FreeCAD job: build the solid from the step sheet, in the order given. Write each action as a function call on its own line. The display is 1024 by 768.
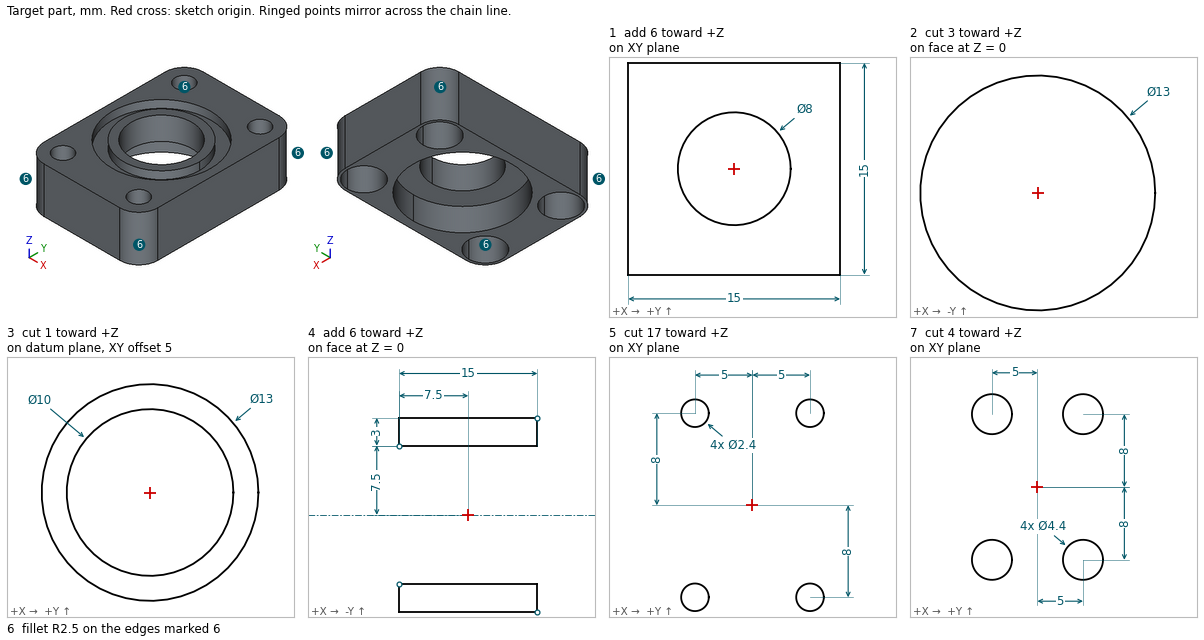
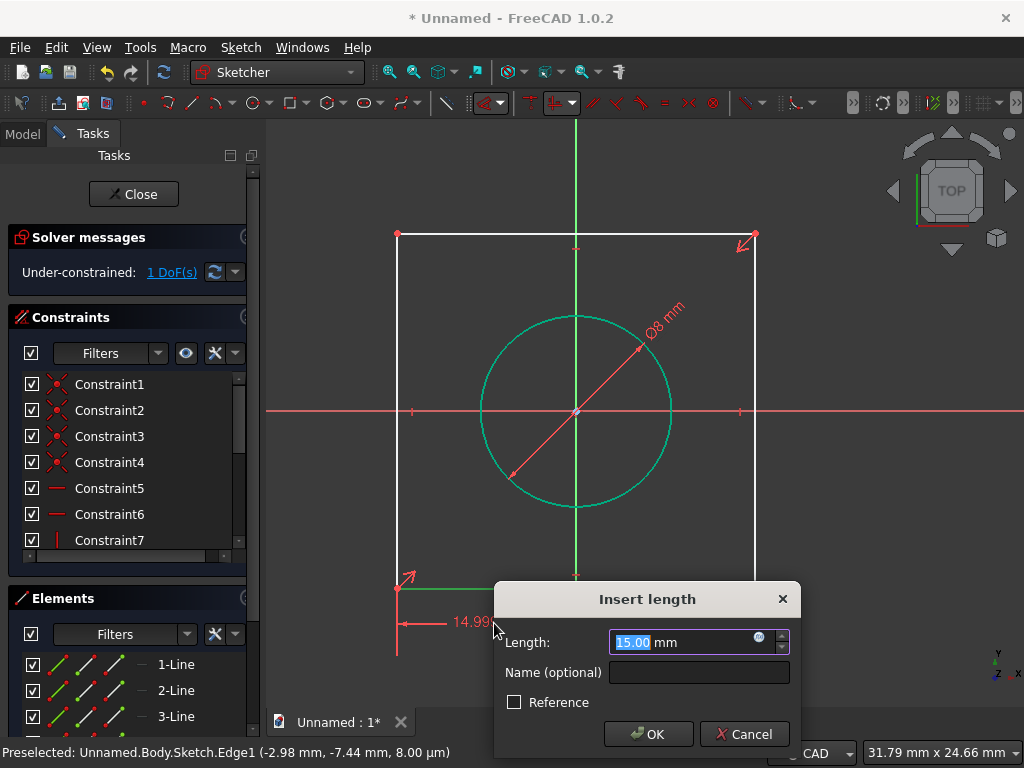
text(15)
key(Return)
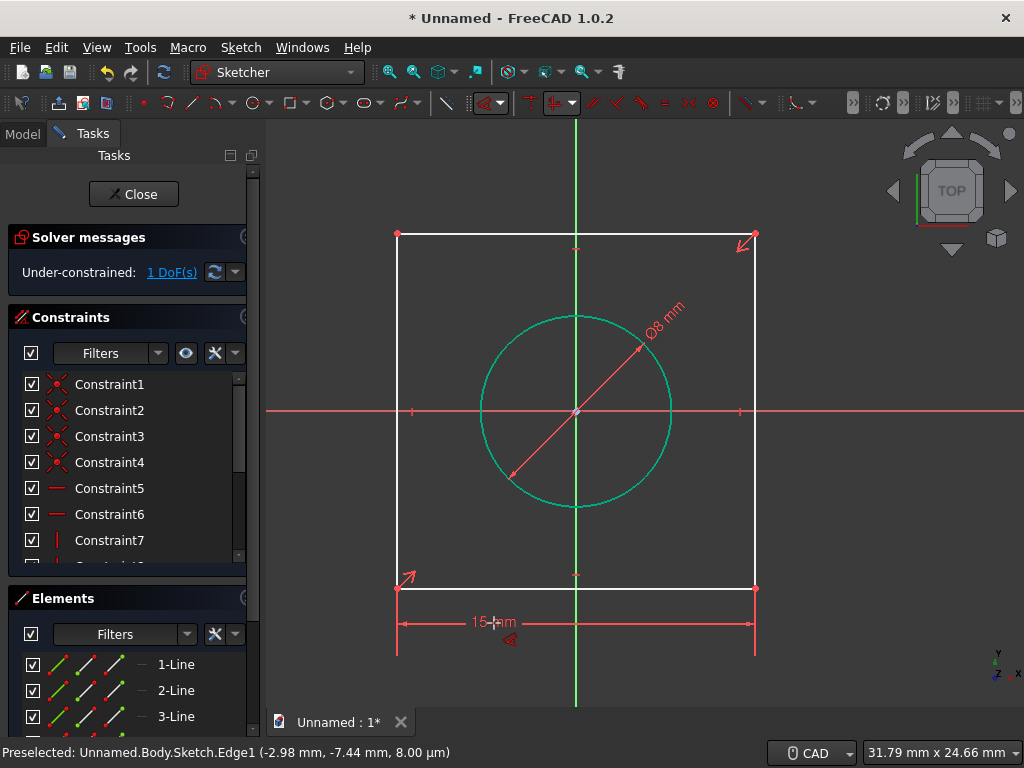
click(755, 482)
click(789, 330)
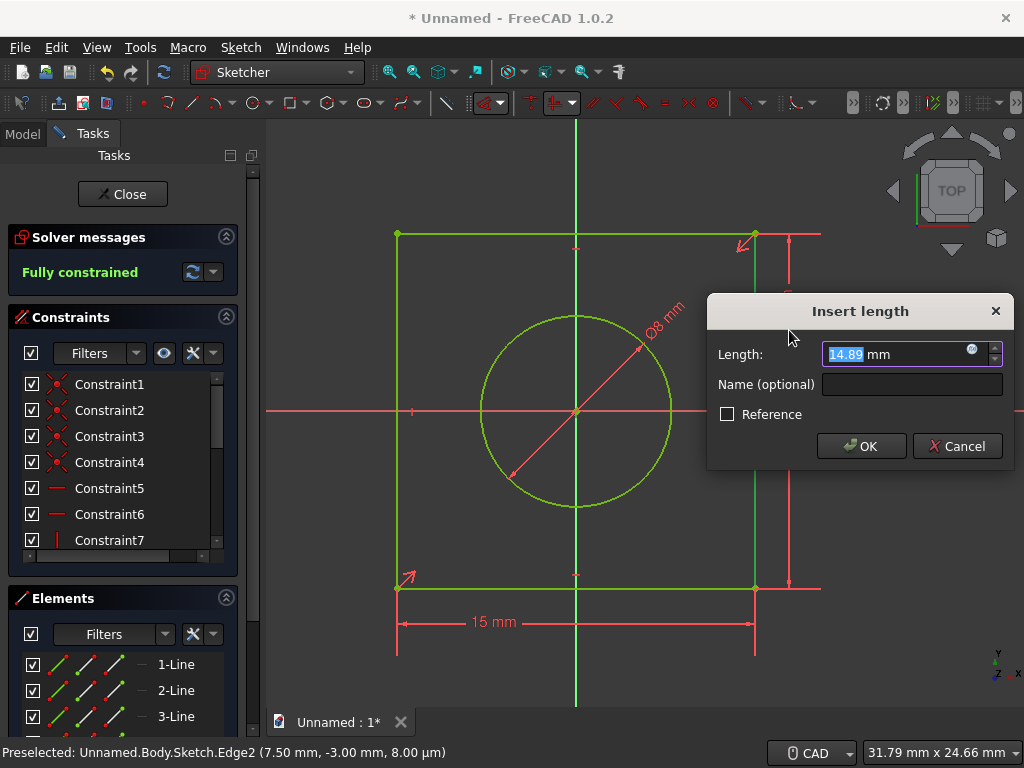
text(15)
key(Return)
key(Escape)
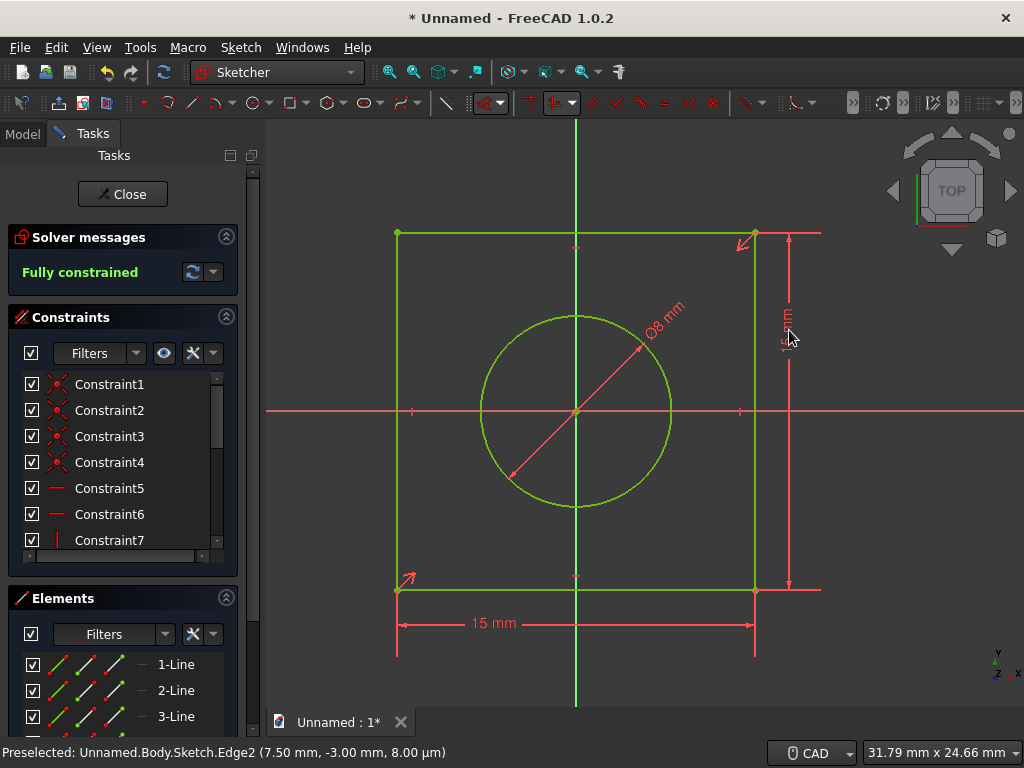
click(123, 194)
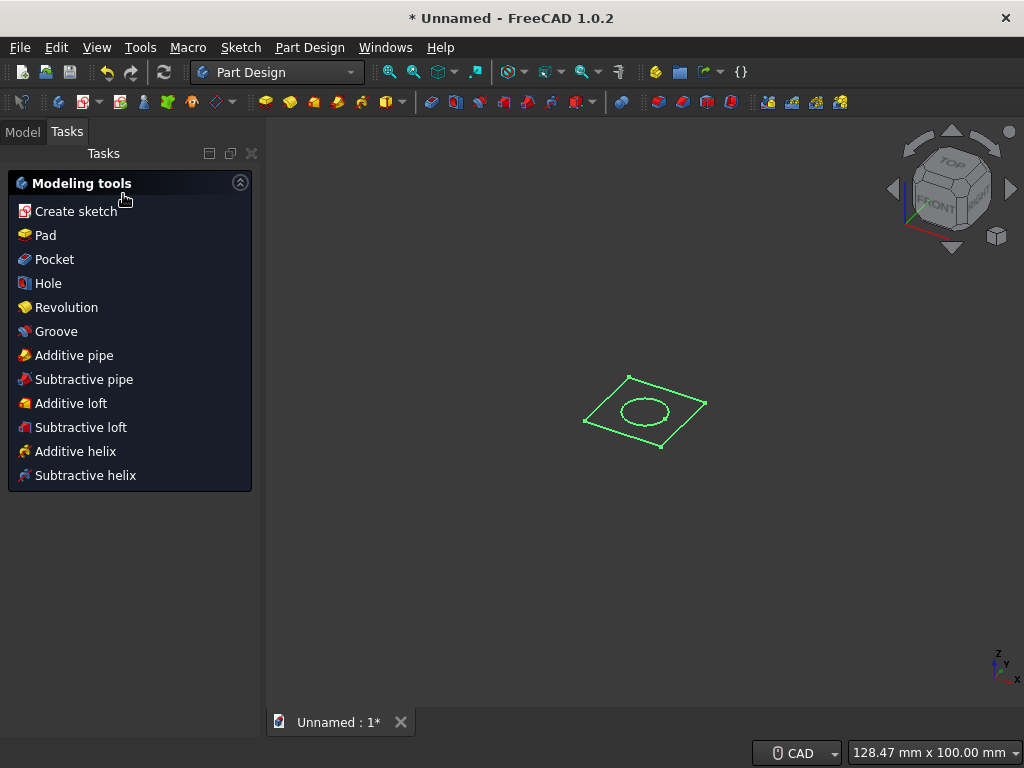
click(266, 102)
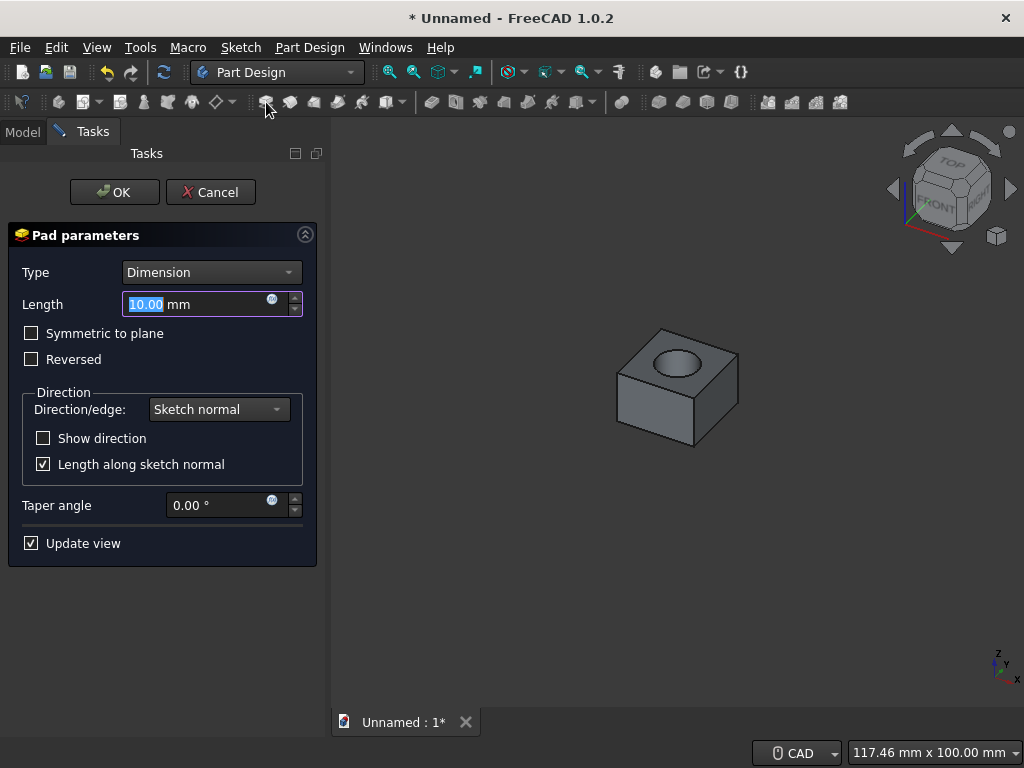
text(6)
key(Tab)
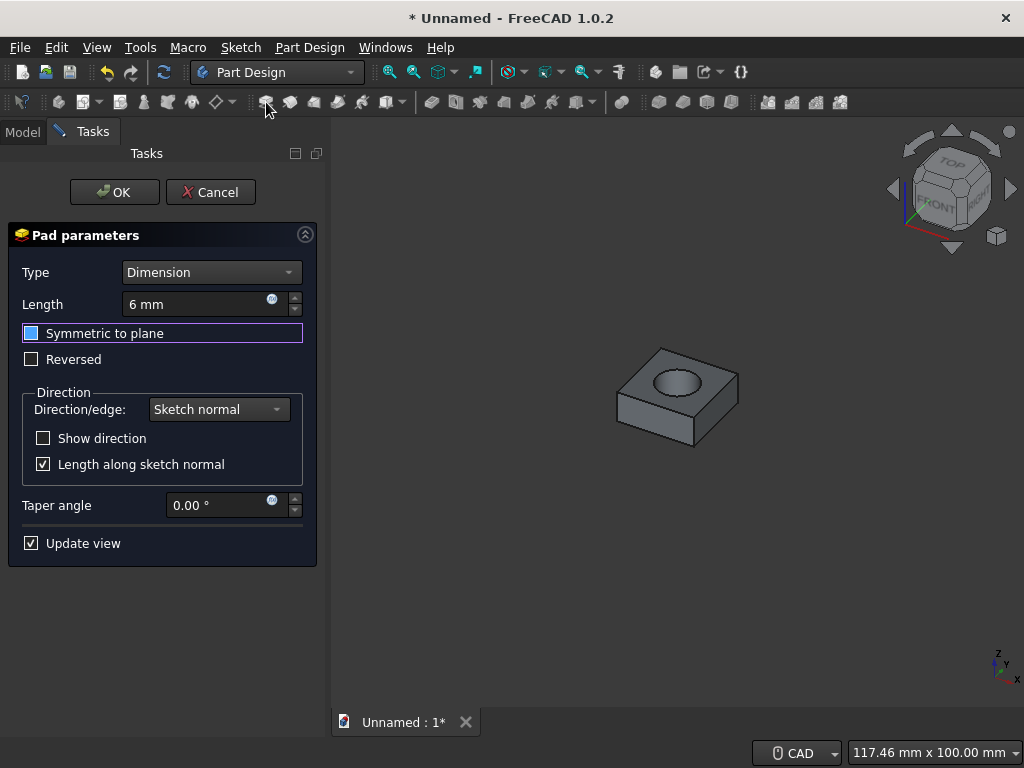
click(115, 192)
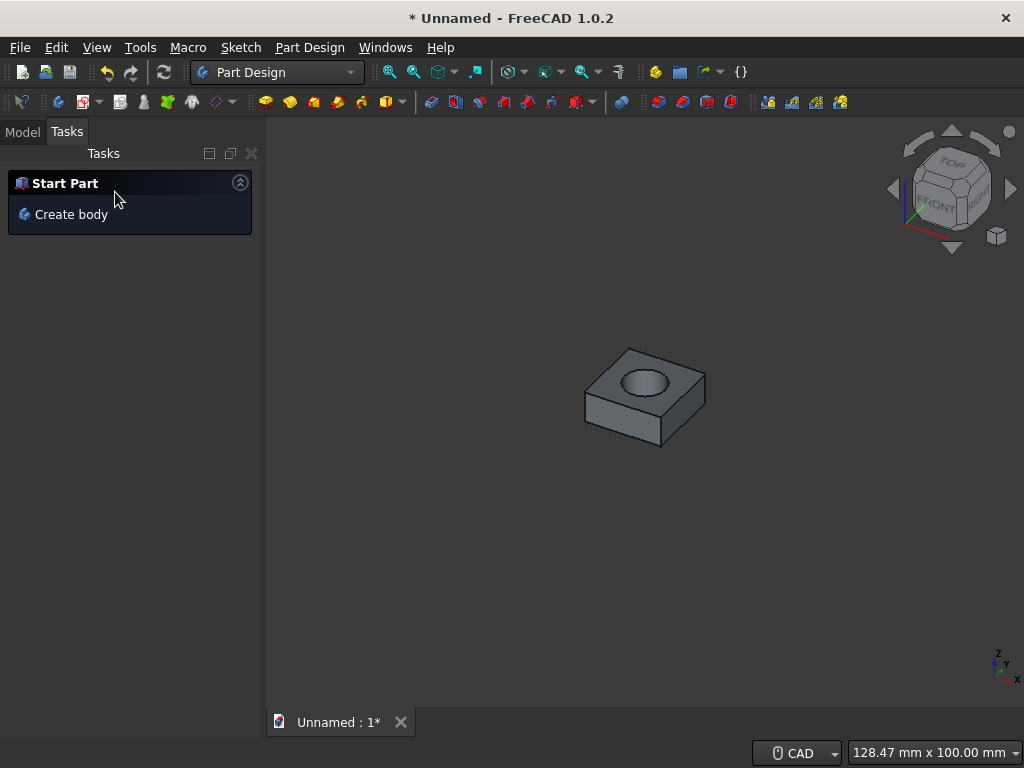
click(390, 72)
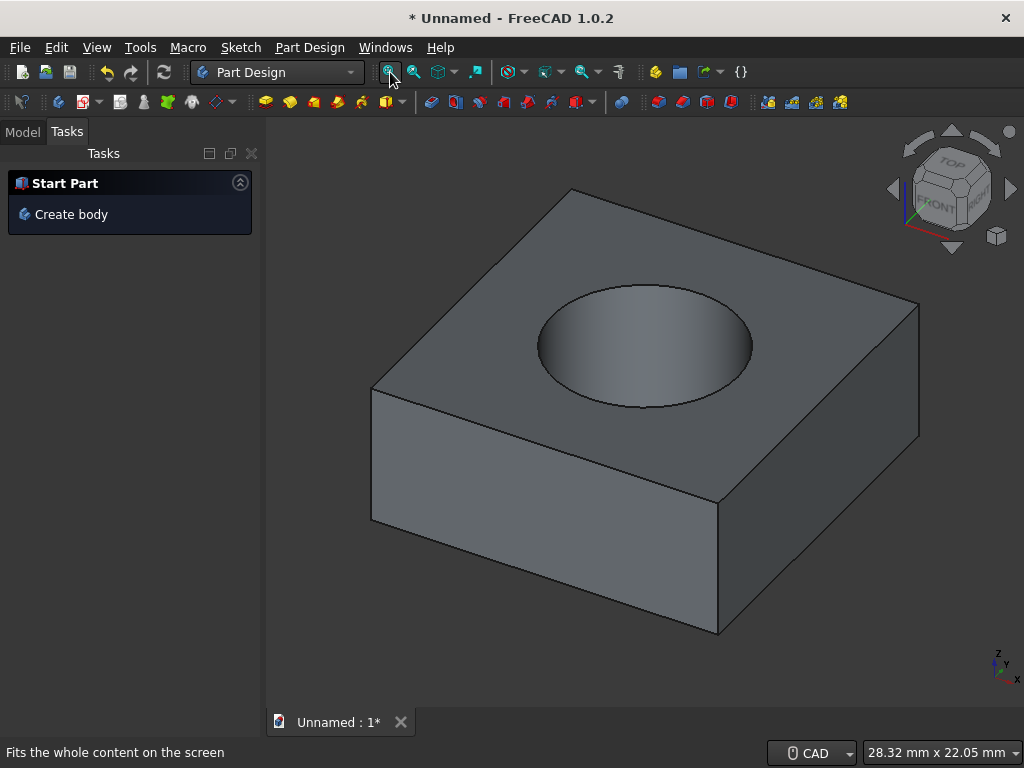
key(5)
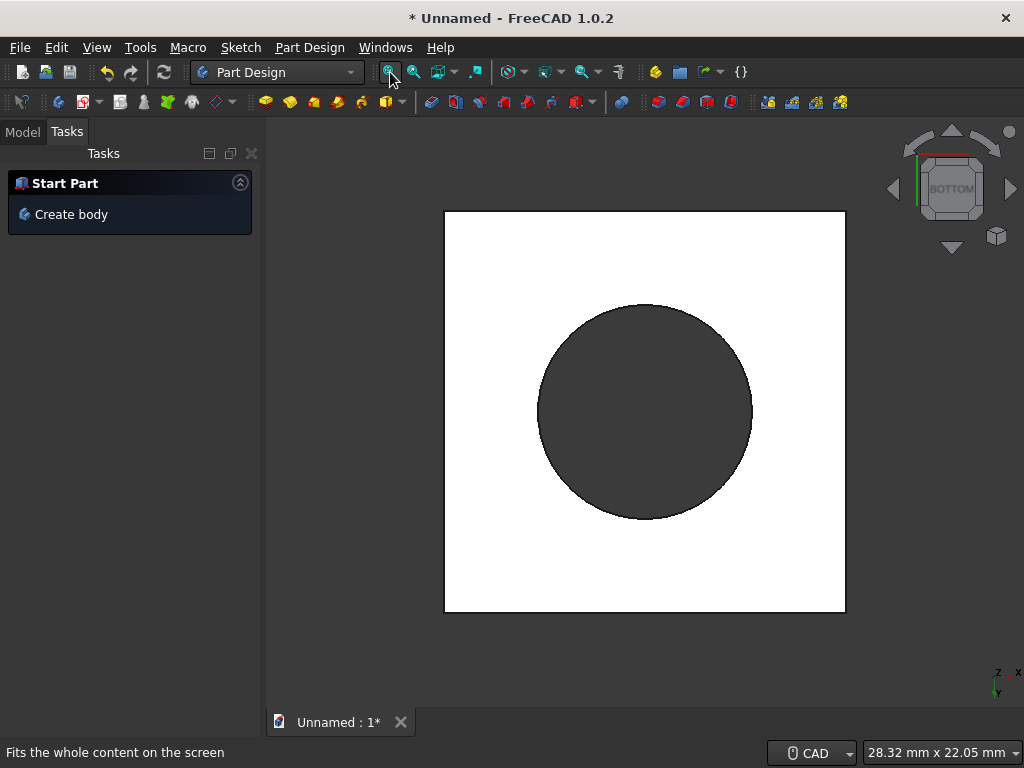
click(760, 526)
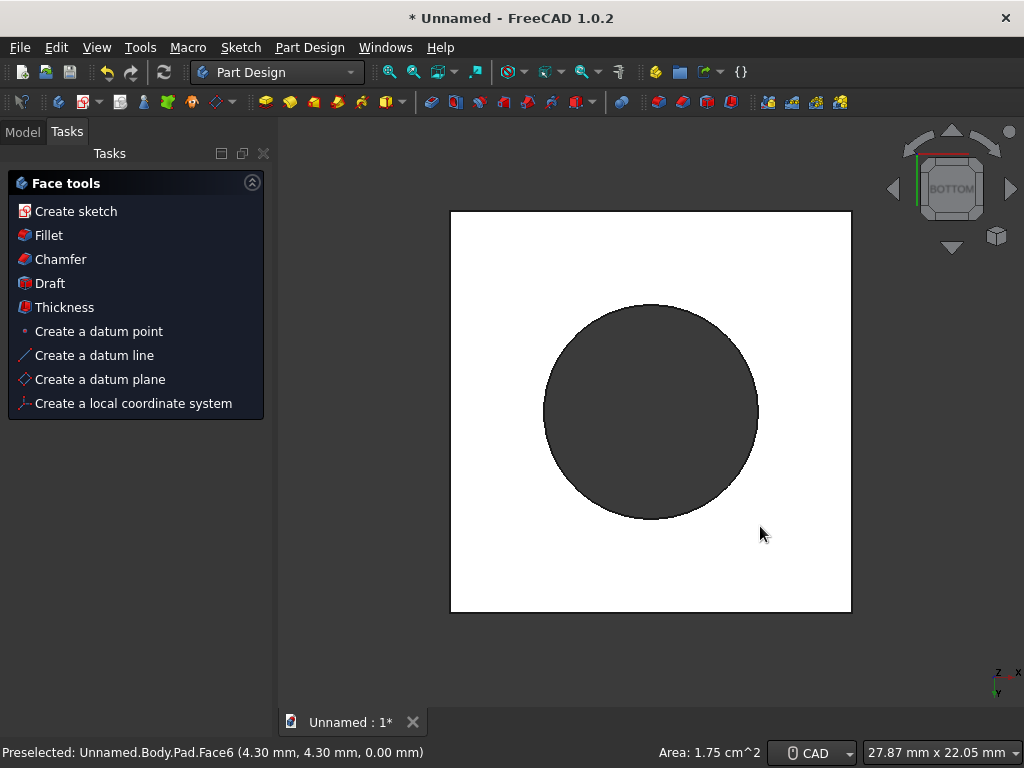
click(84, 102)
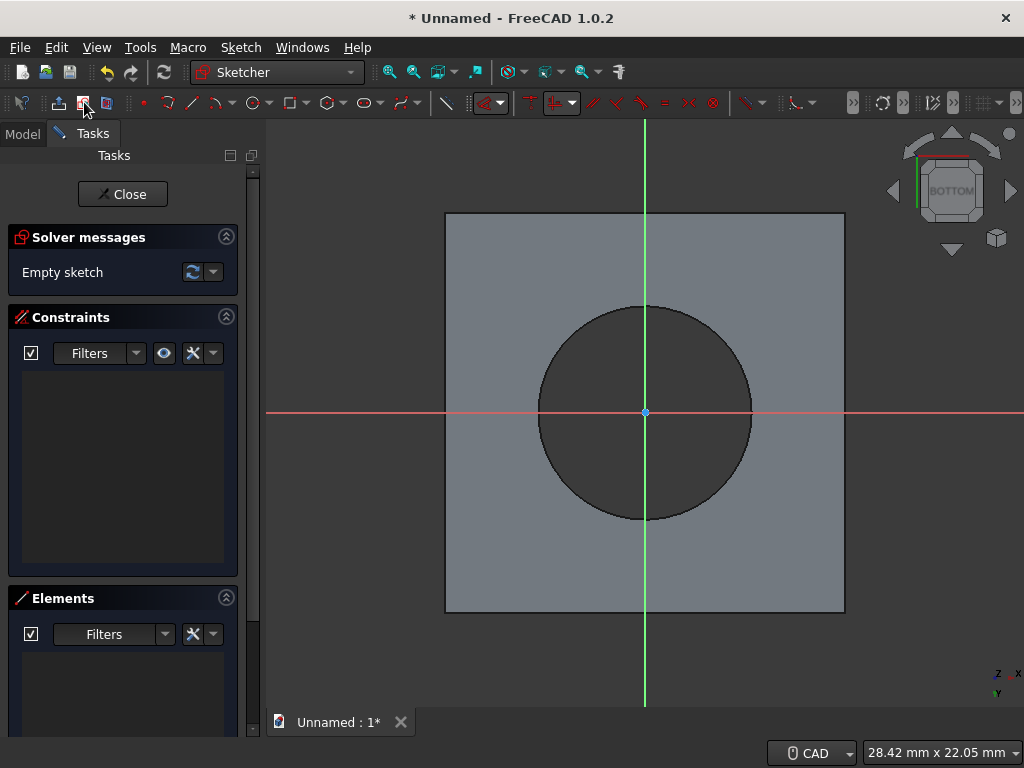
click(254, 104)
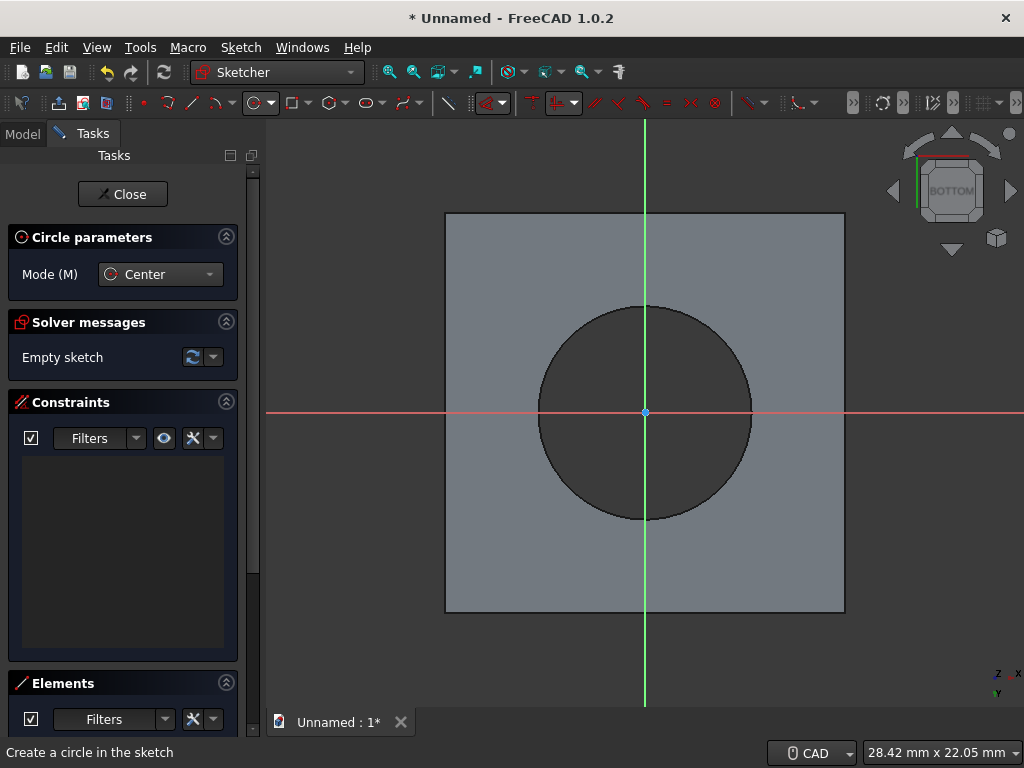
click(645, 413)
click(768, 290)
key(Escape)